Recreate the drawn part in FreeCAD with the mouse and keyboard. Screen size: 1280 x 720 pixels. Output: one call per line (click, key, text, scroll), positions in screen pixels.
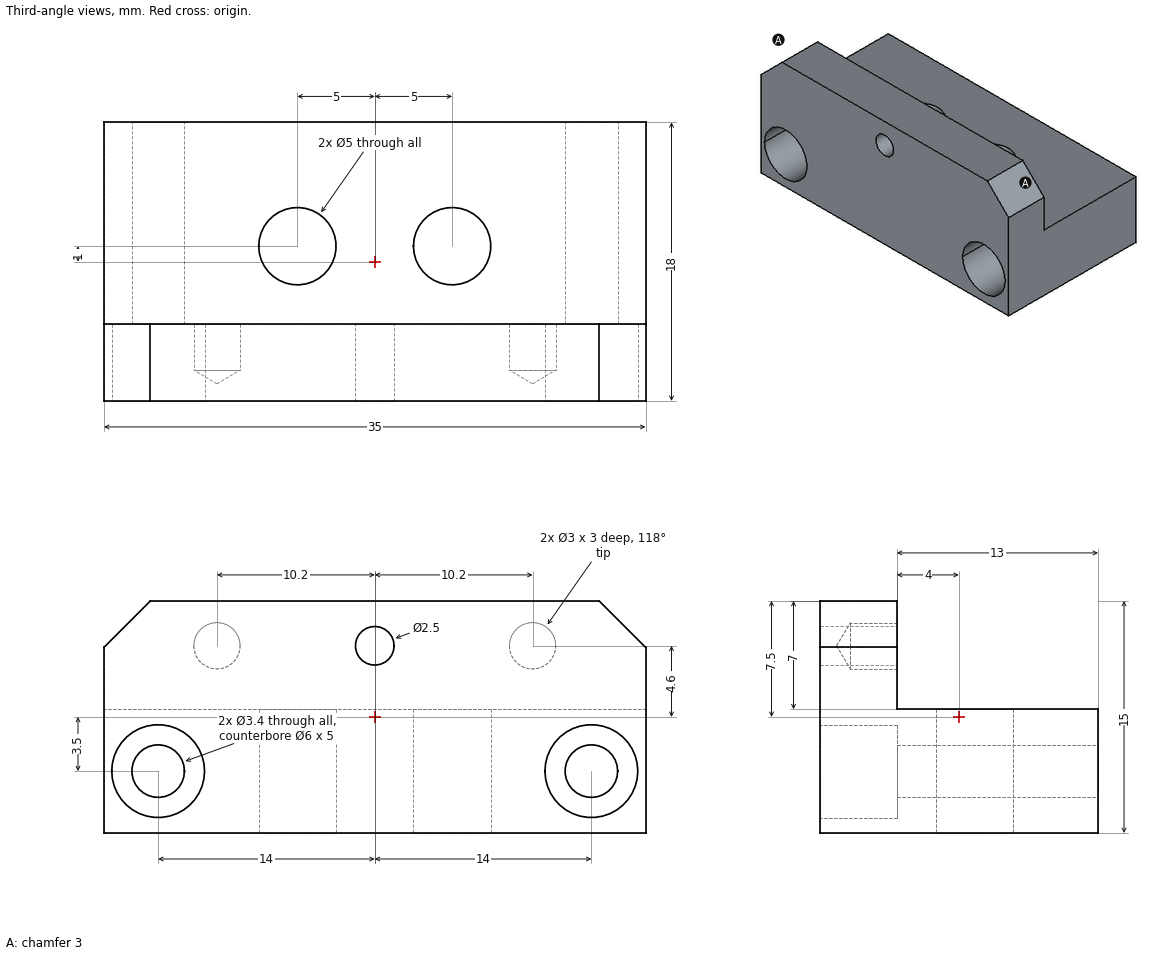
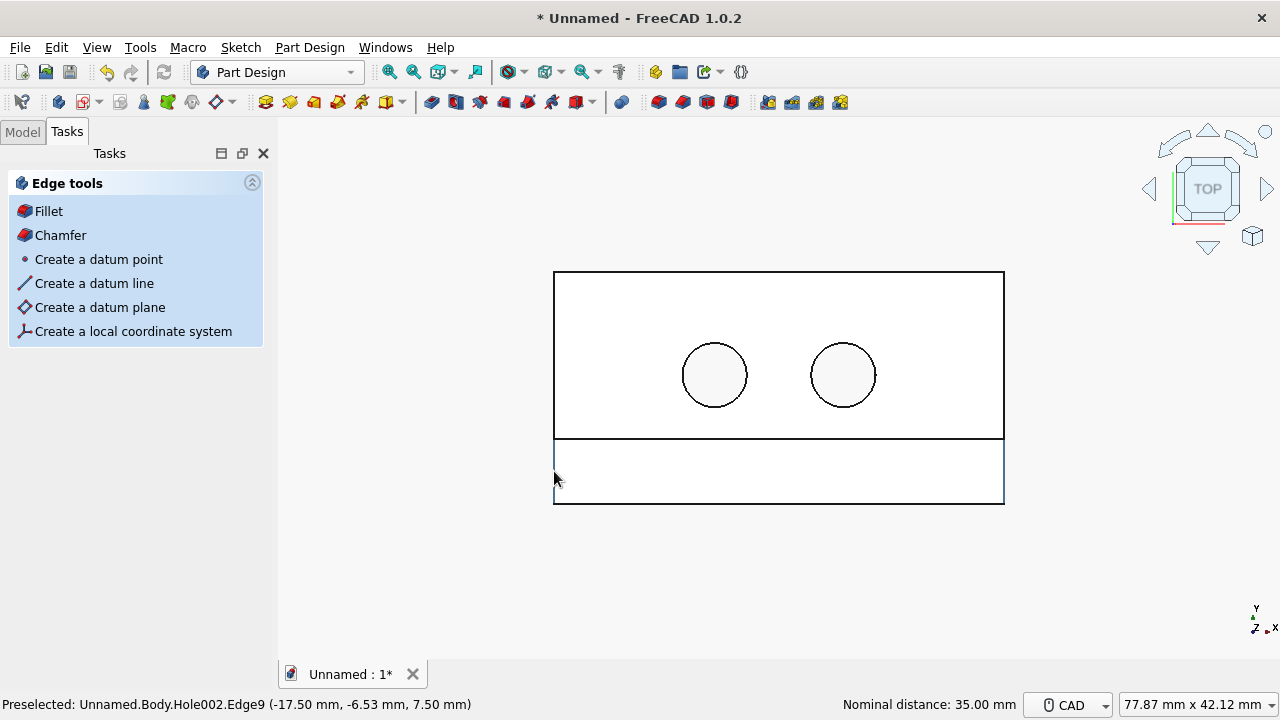
click(684, 102)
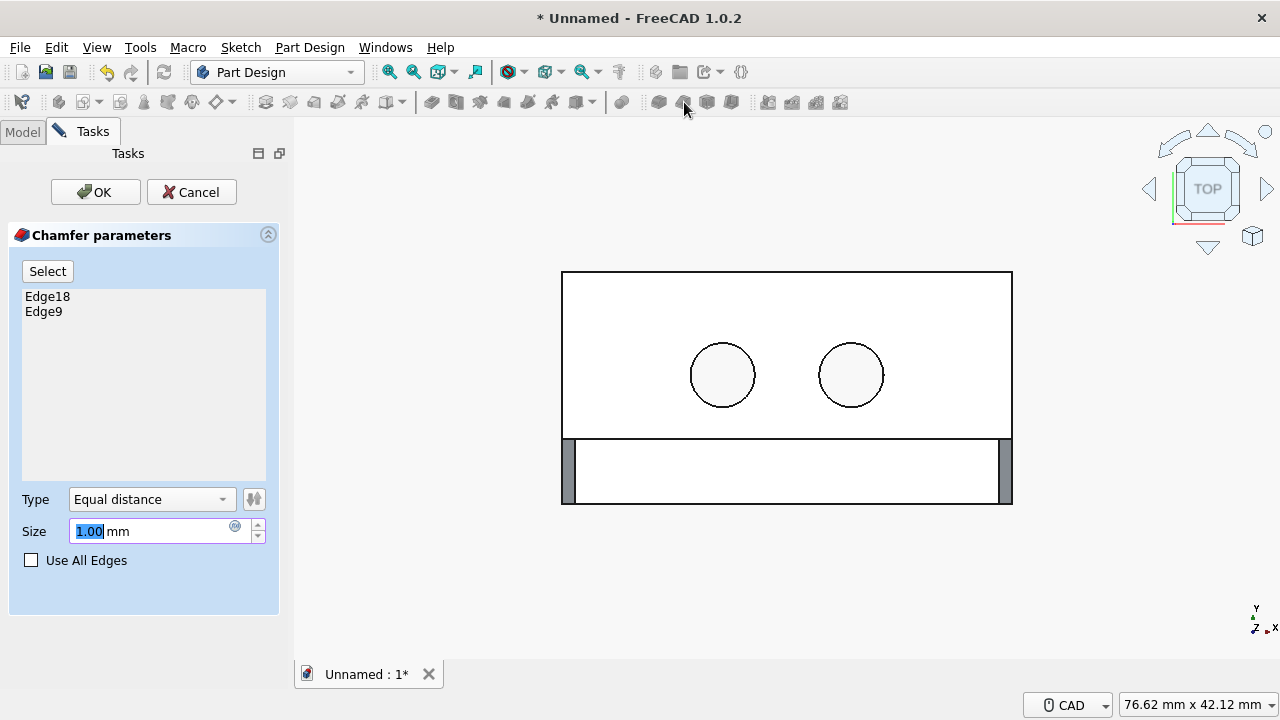
text(3)
key(Tab)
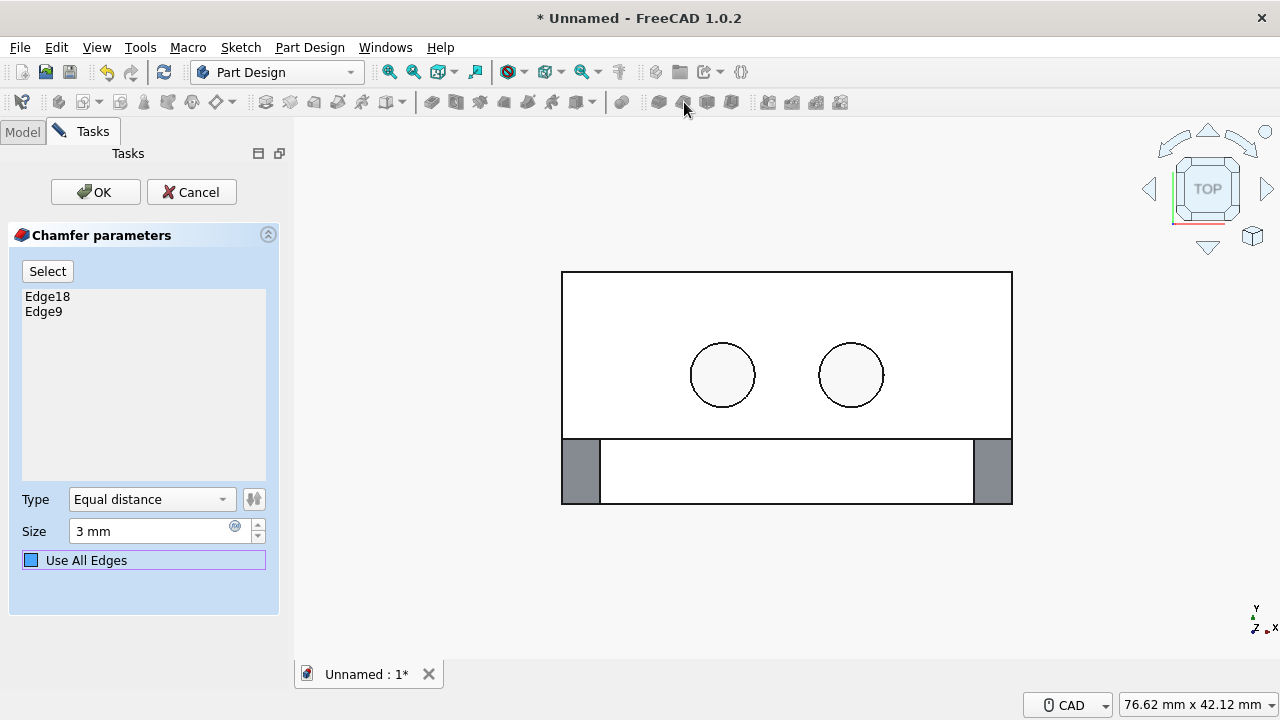
click(96, 192)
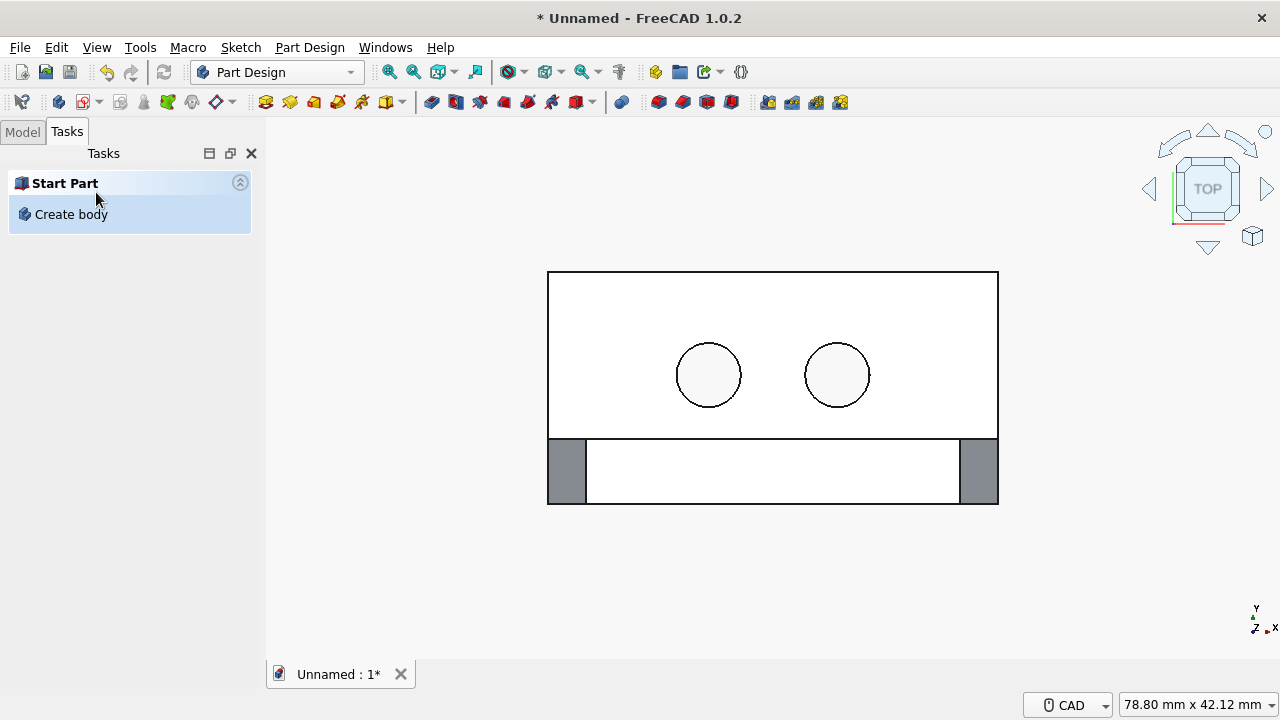
key(0)